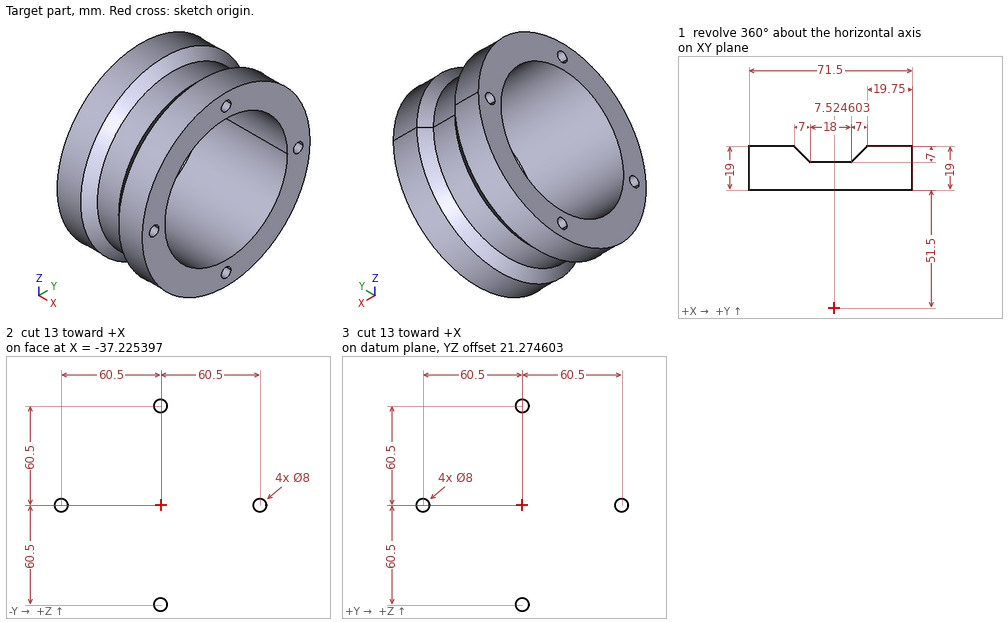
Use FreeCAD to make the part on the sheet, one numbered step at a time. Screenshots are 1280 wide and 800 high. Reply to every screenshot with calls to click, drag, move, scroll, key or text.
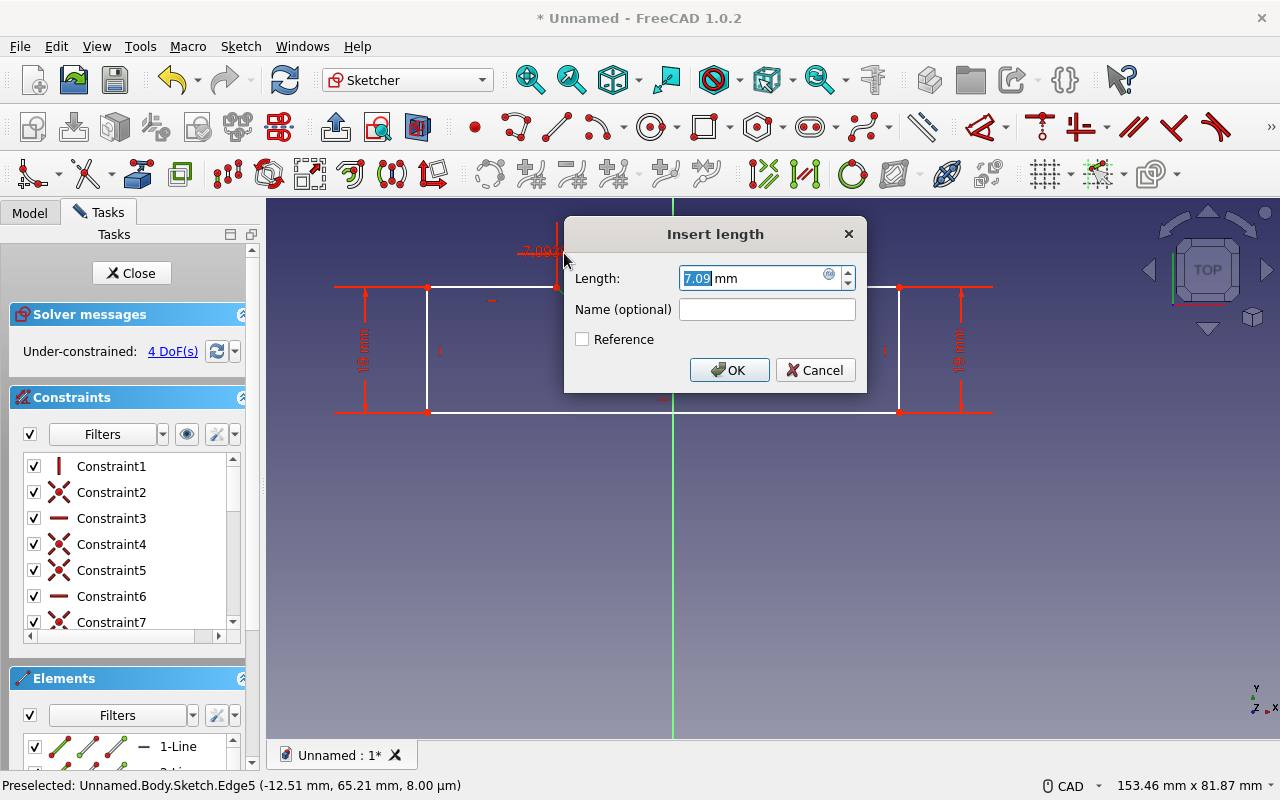
text(7)
key(Return)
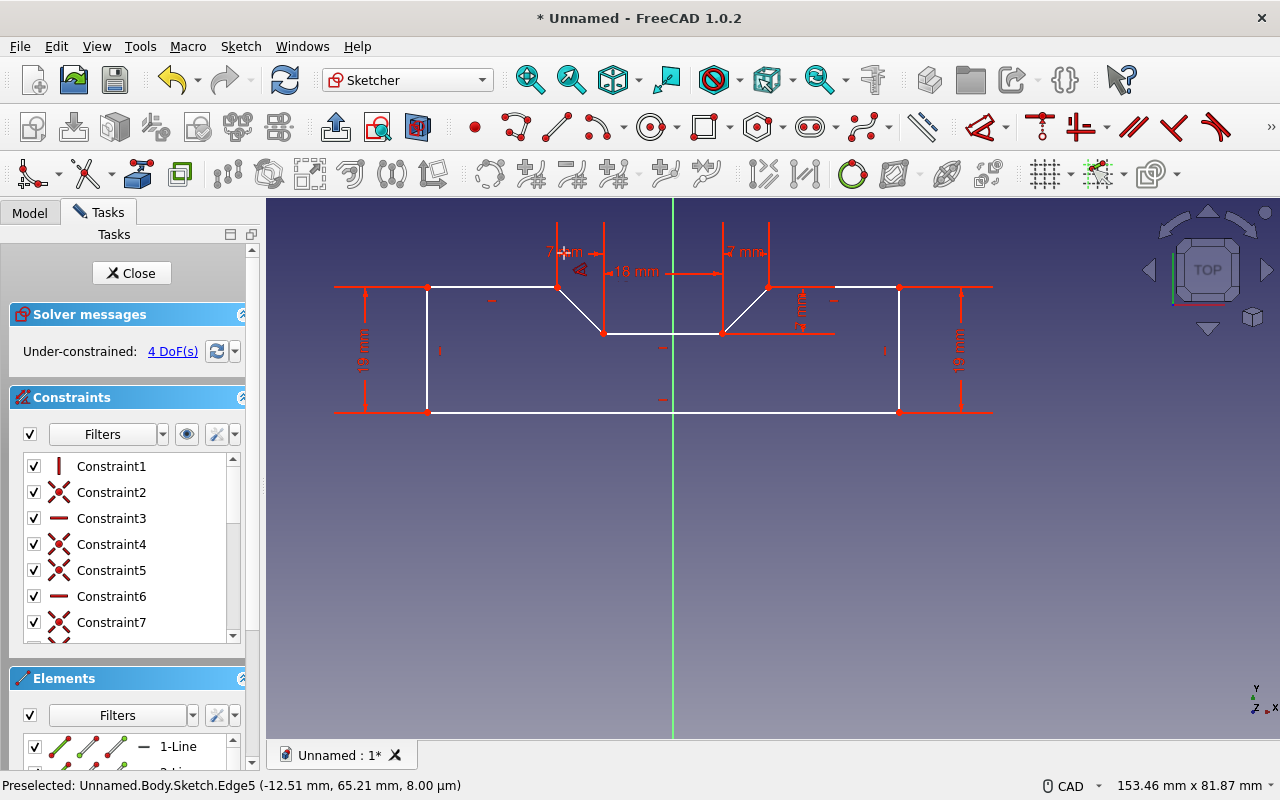
click(569, 413)
click(555, 379)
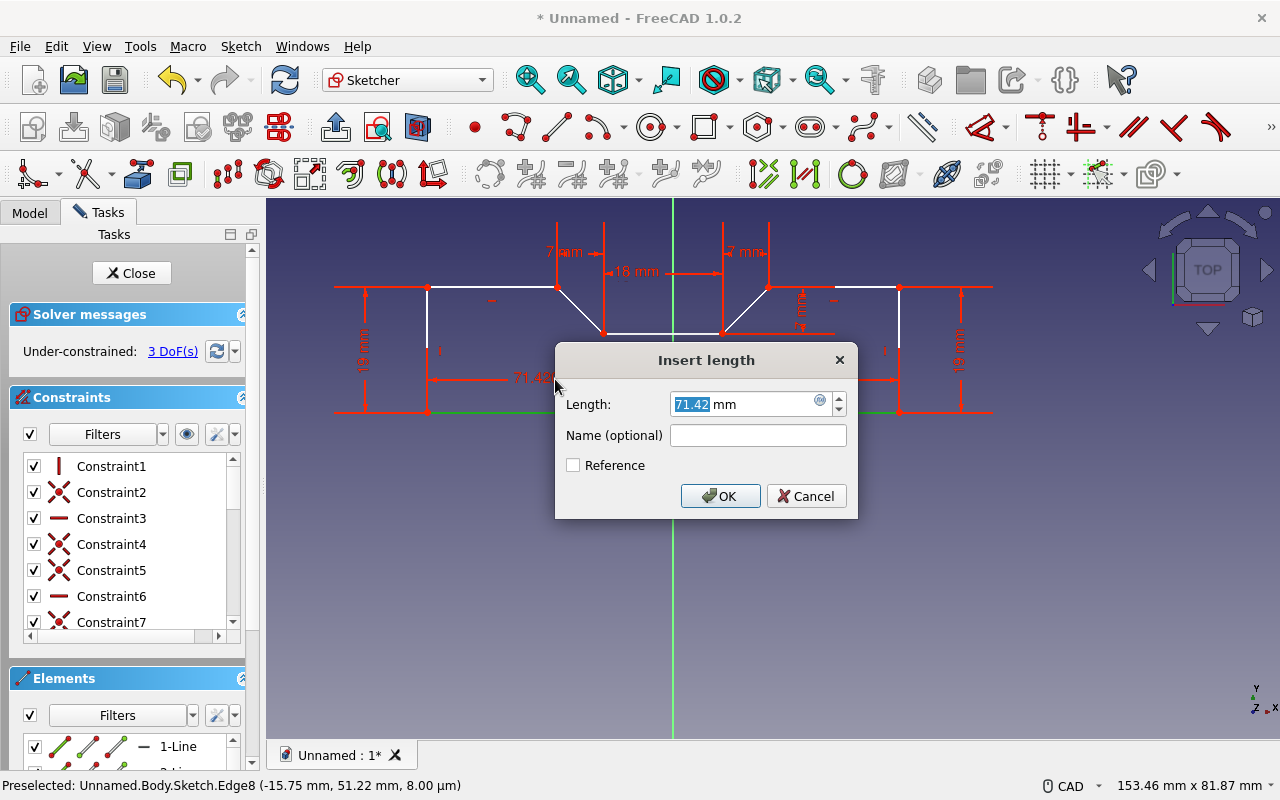
text(71.5)
key(Return)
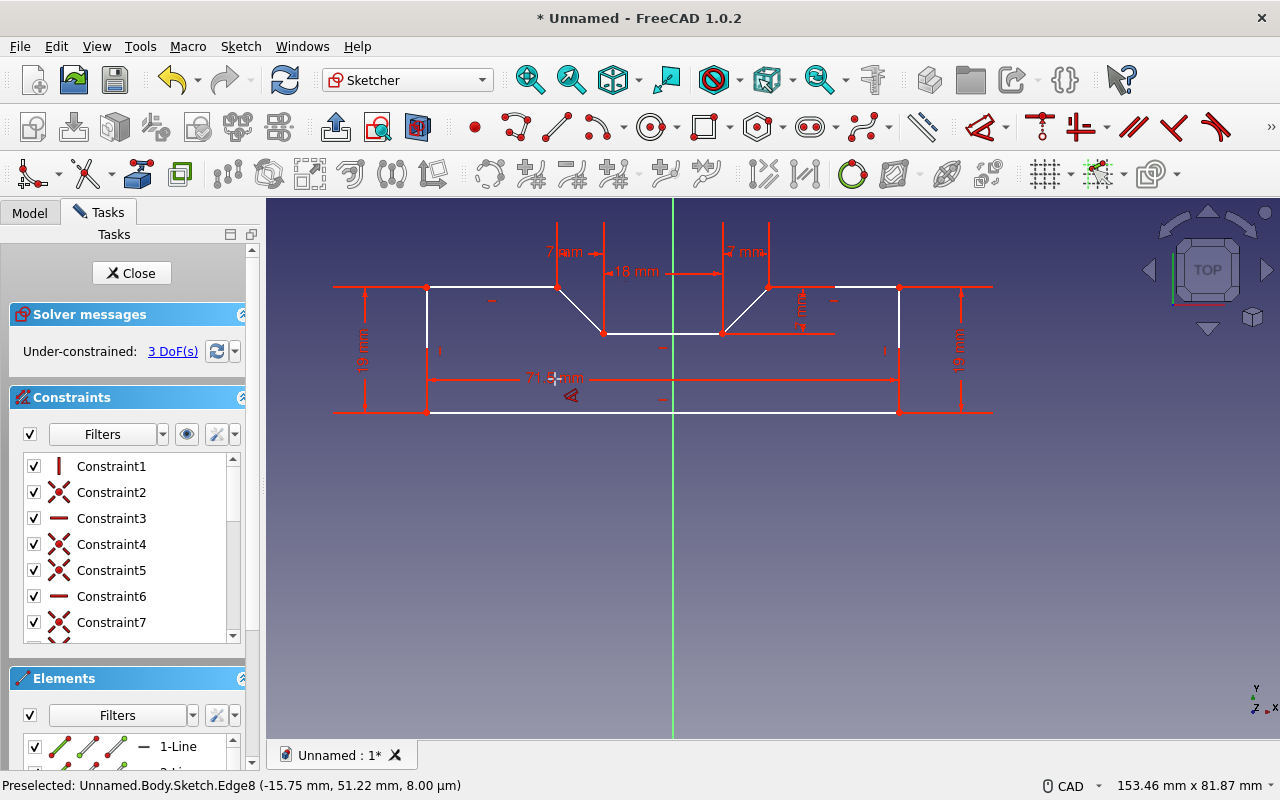
click(860, 287)
click(834, 253)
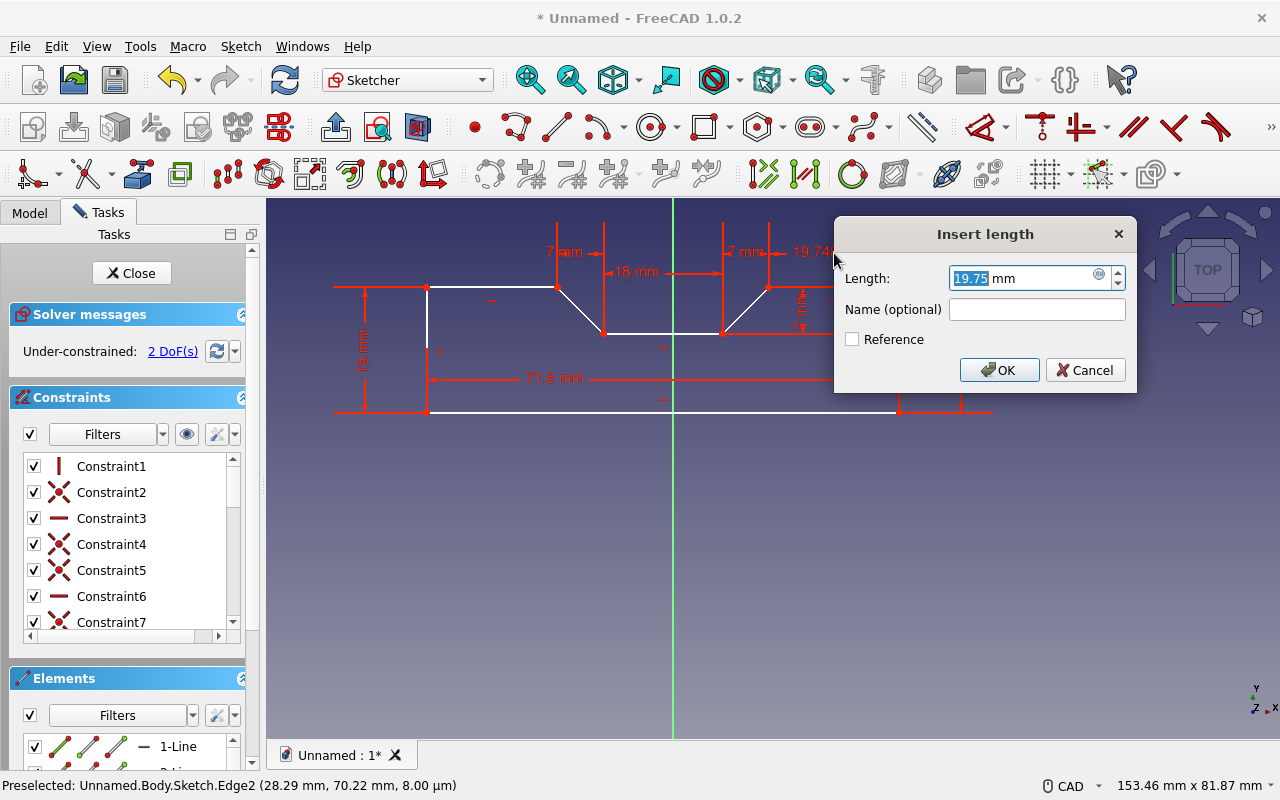
text(19.75)
key(Return)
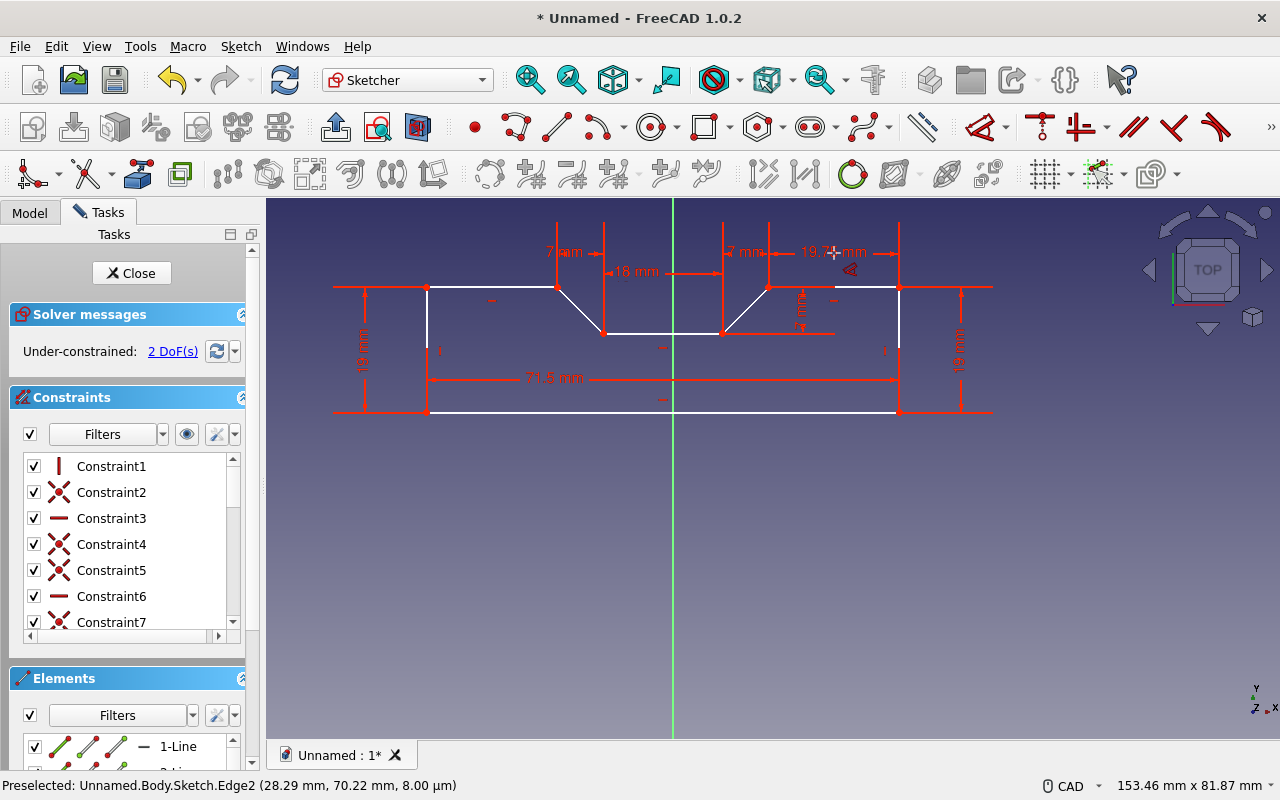
click(899, 413)
click(933, 562)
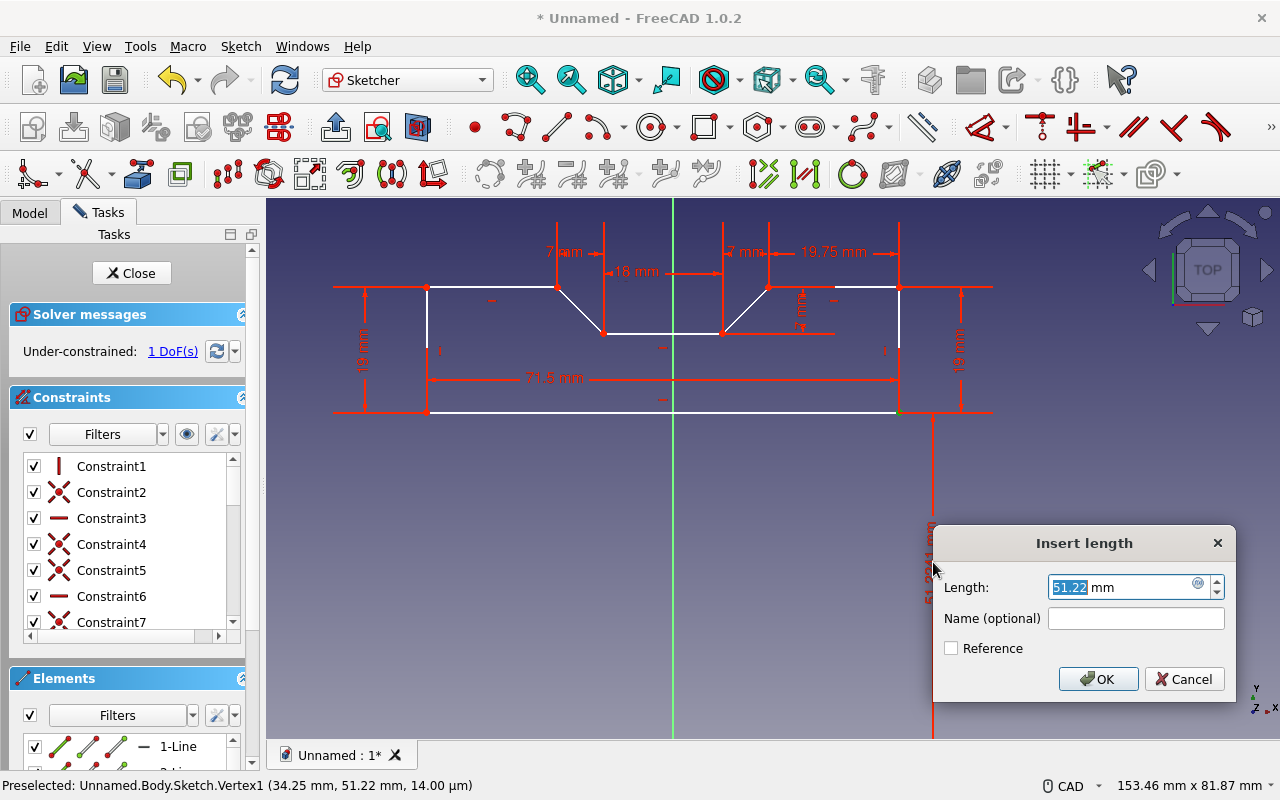
text(51.5)
key(Return)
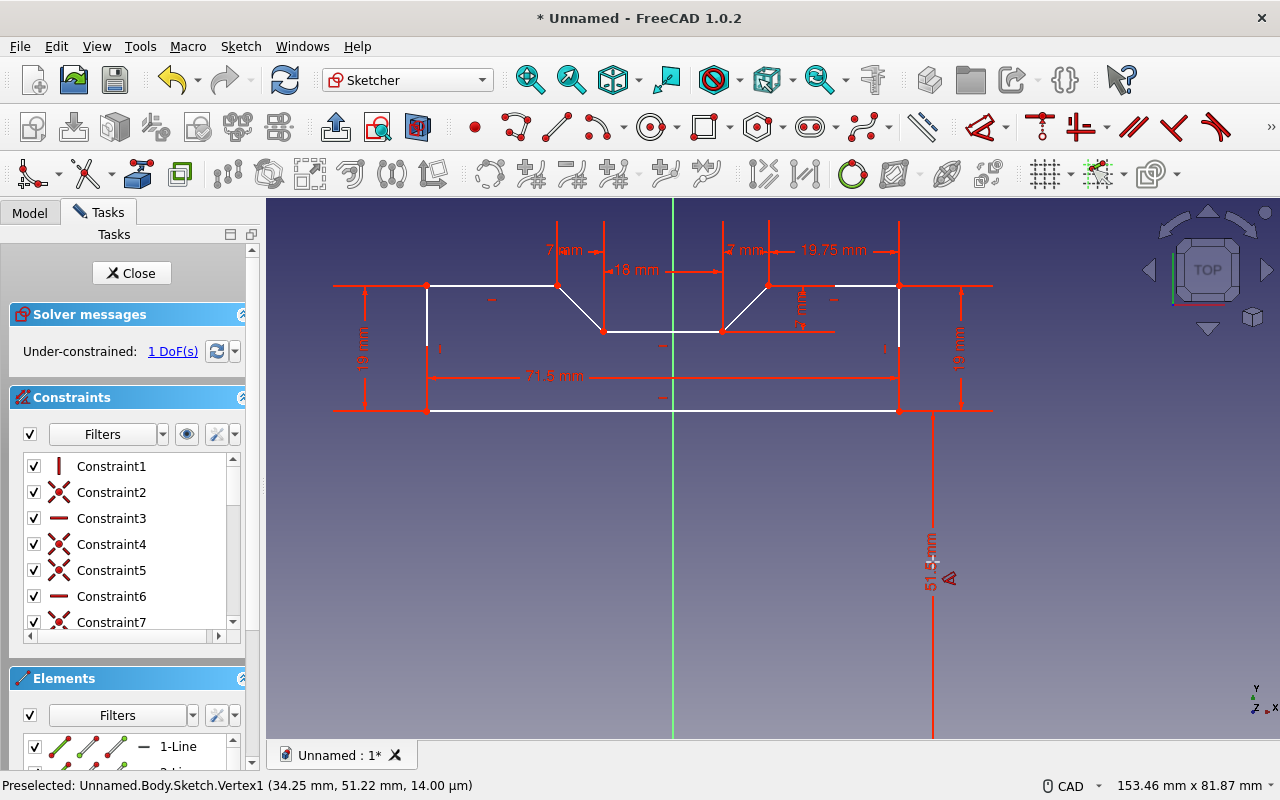
click(723, 332)
click(698, 298)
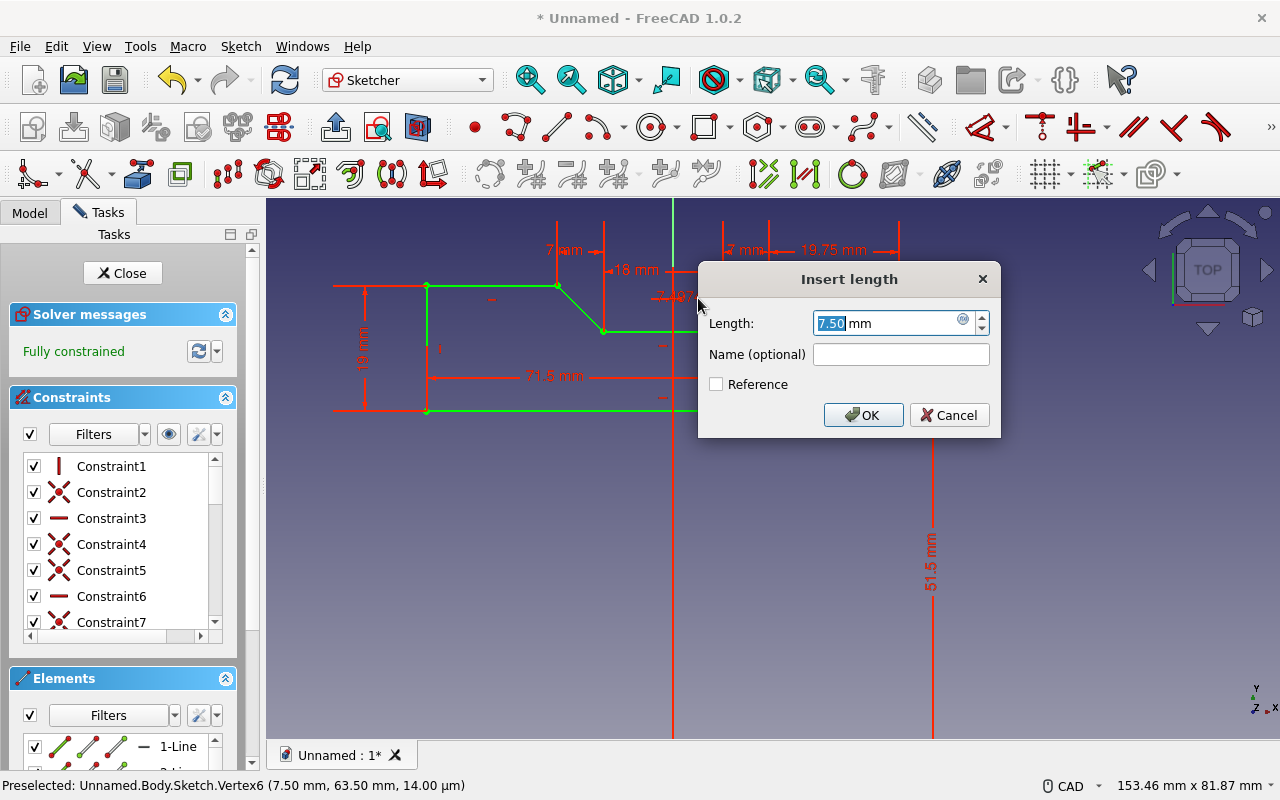
text(7.524603)
key(Return)
key(Escape)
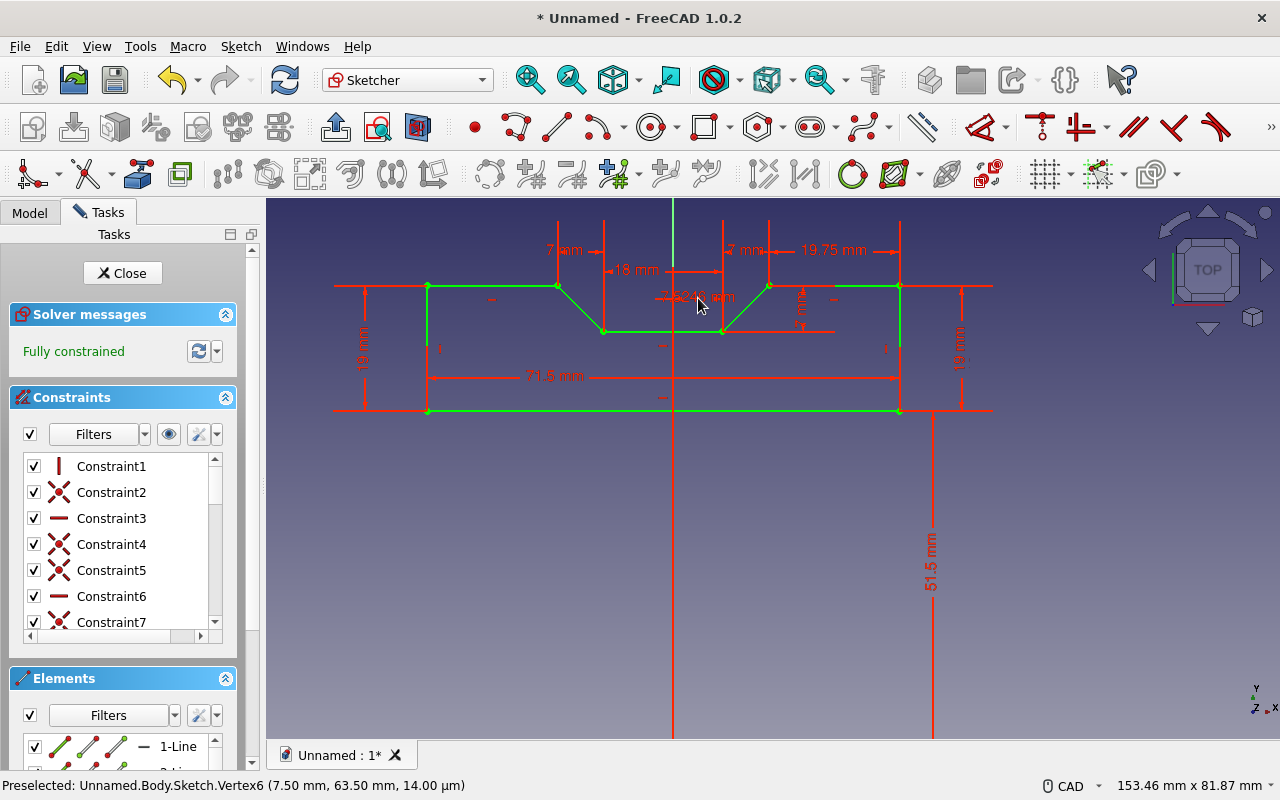
click(123, 273)